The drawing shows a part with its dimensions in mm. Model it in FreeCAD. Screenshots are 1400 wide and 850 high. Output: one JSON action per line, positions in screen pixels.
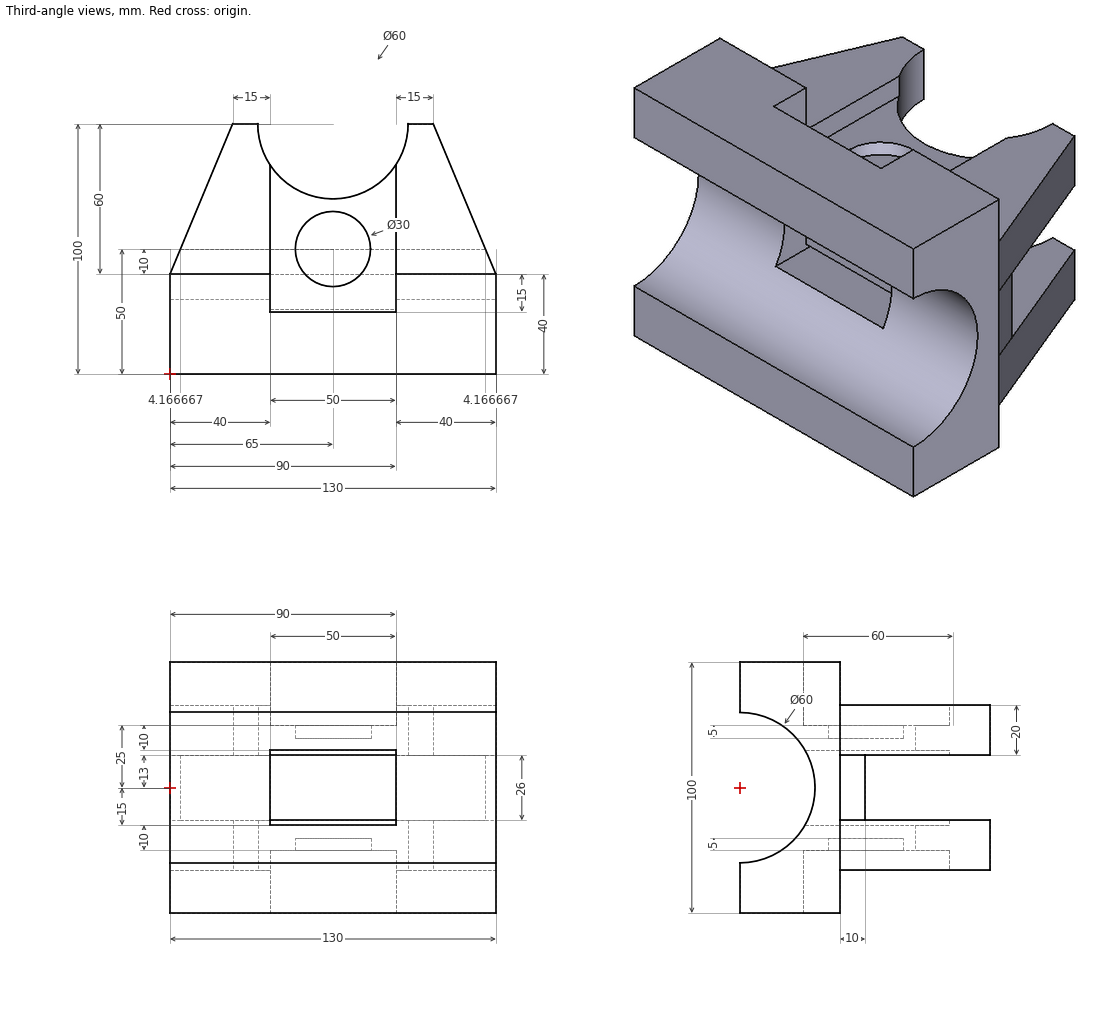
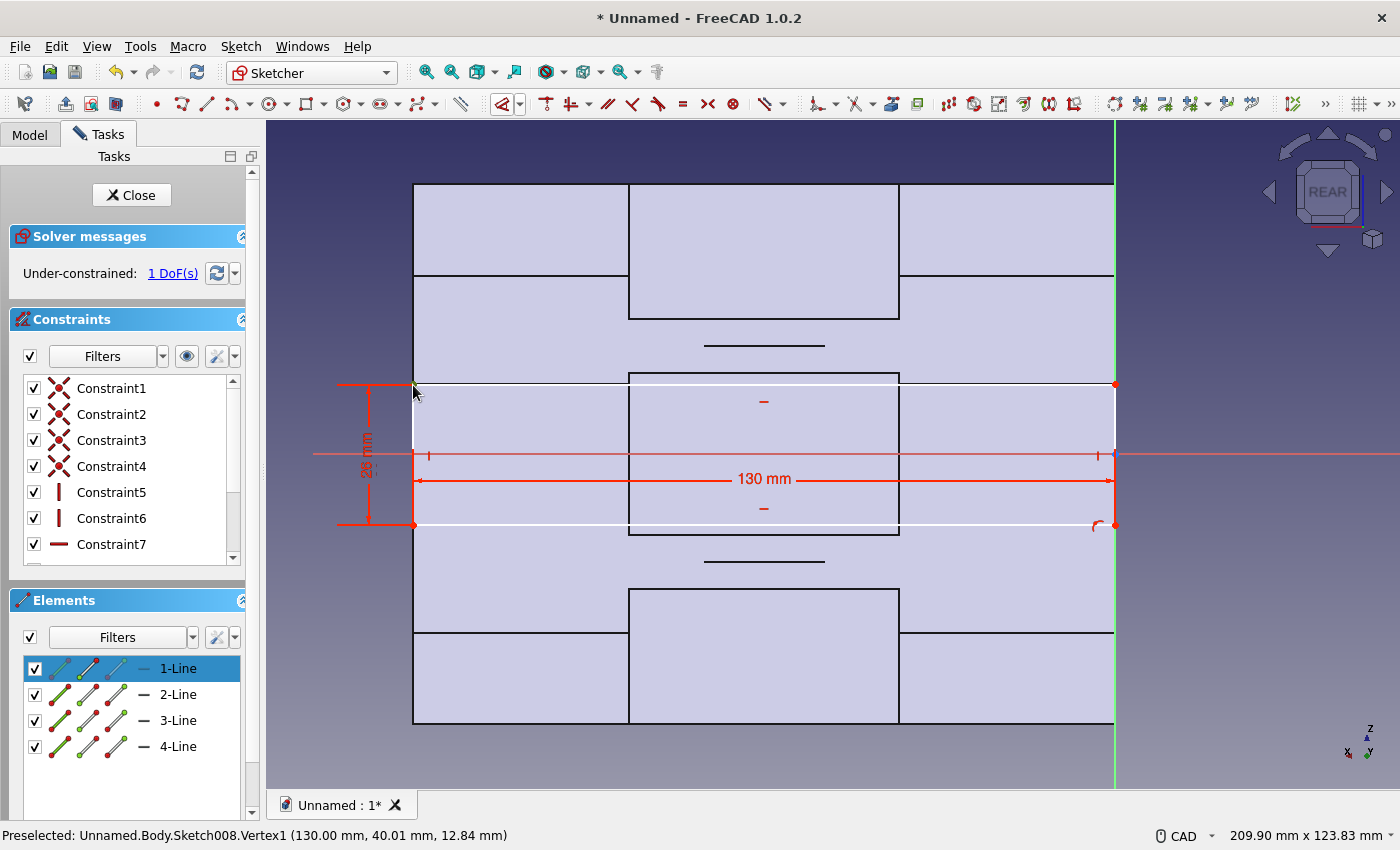
{"action": "left_click", "coordinate": [520, 104]}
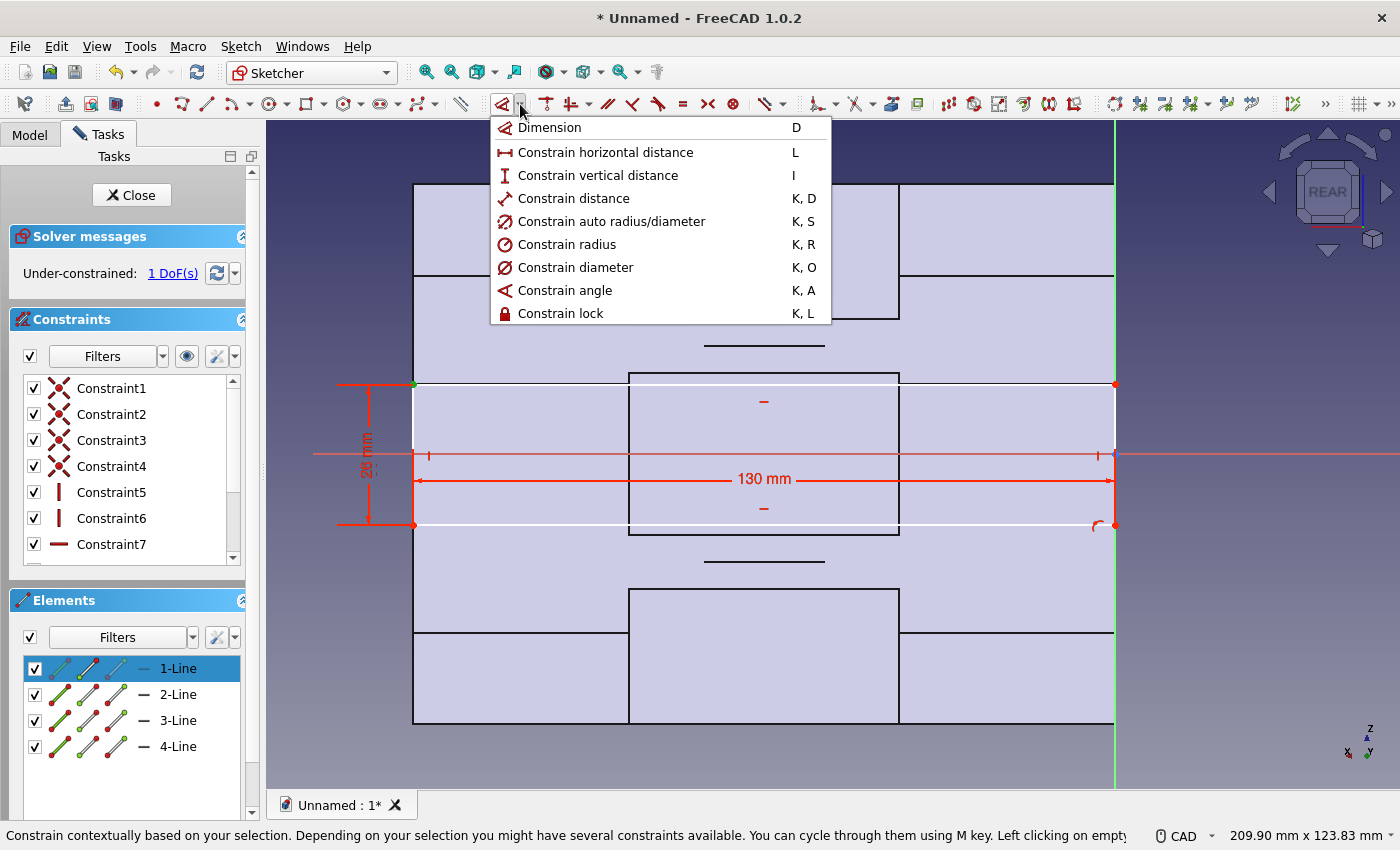
{"action": "left_click", "coordinate": [661, 176]}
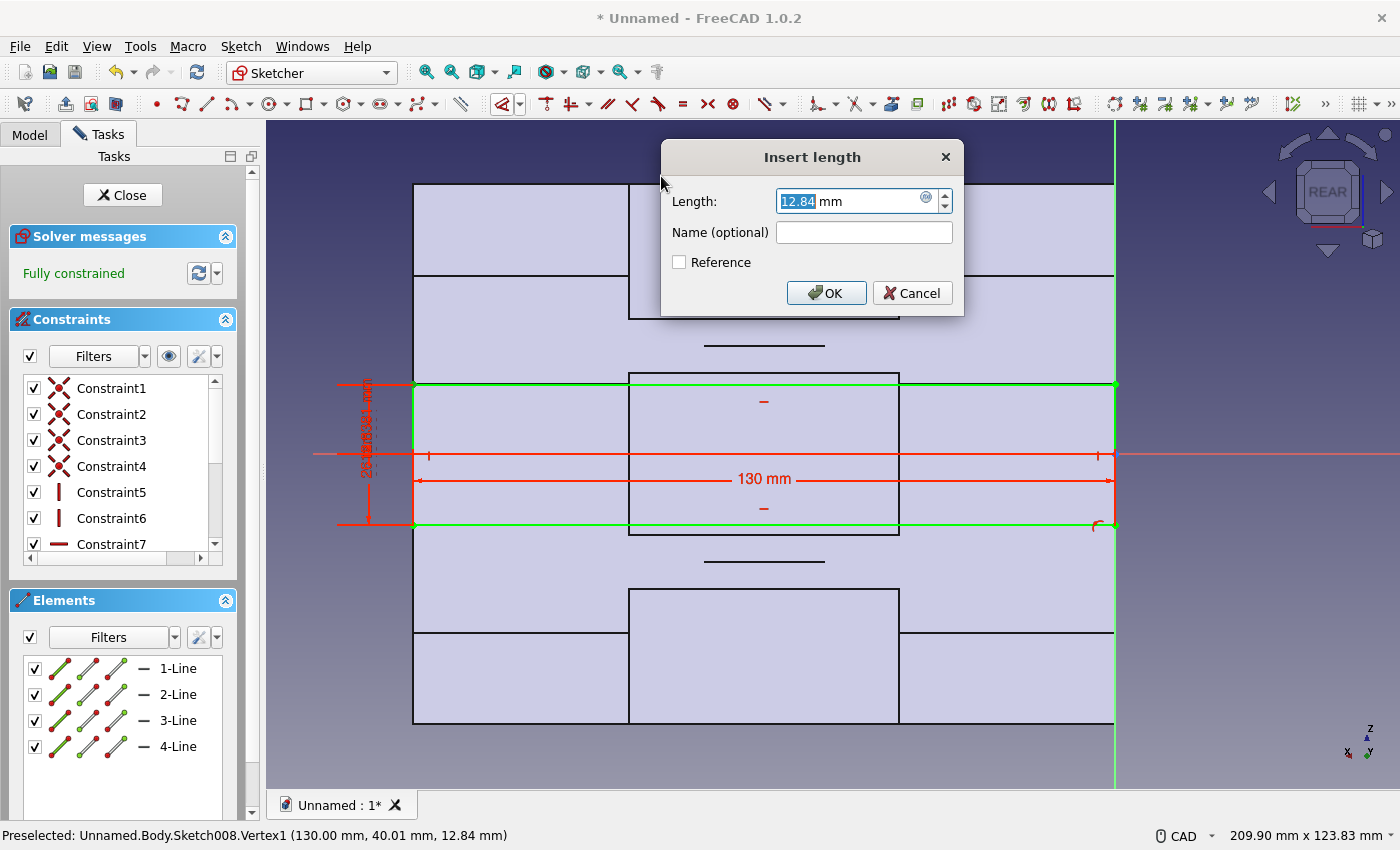
{"action": "type", "text": "13"}
{"action": "key", "text": "Return"}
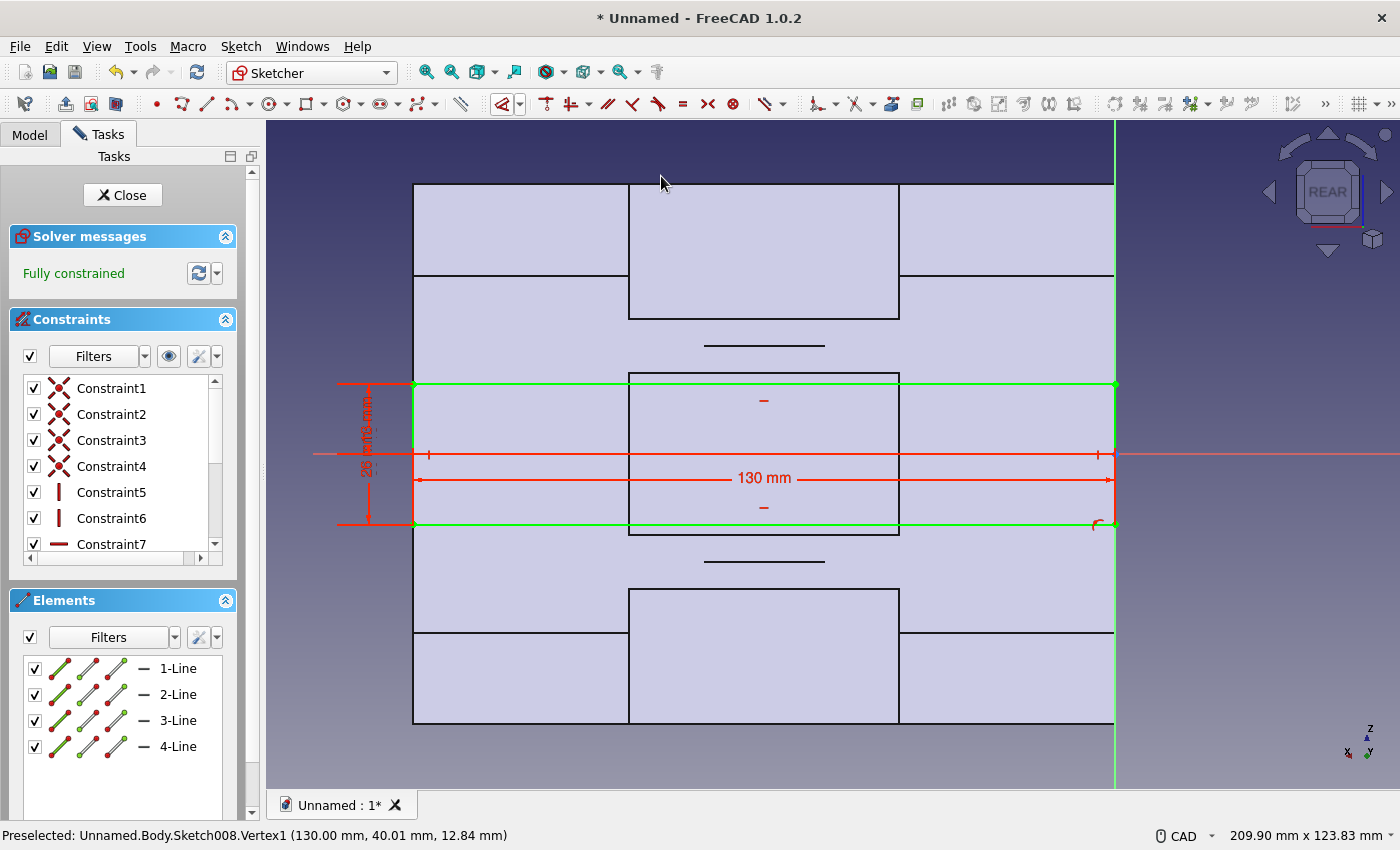
{"action": "left_click", "coordinate": [123, 195]}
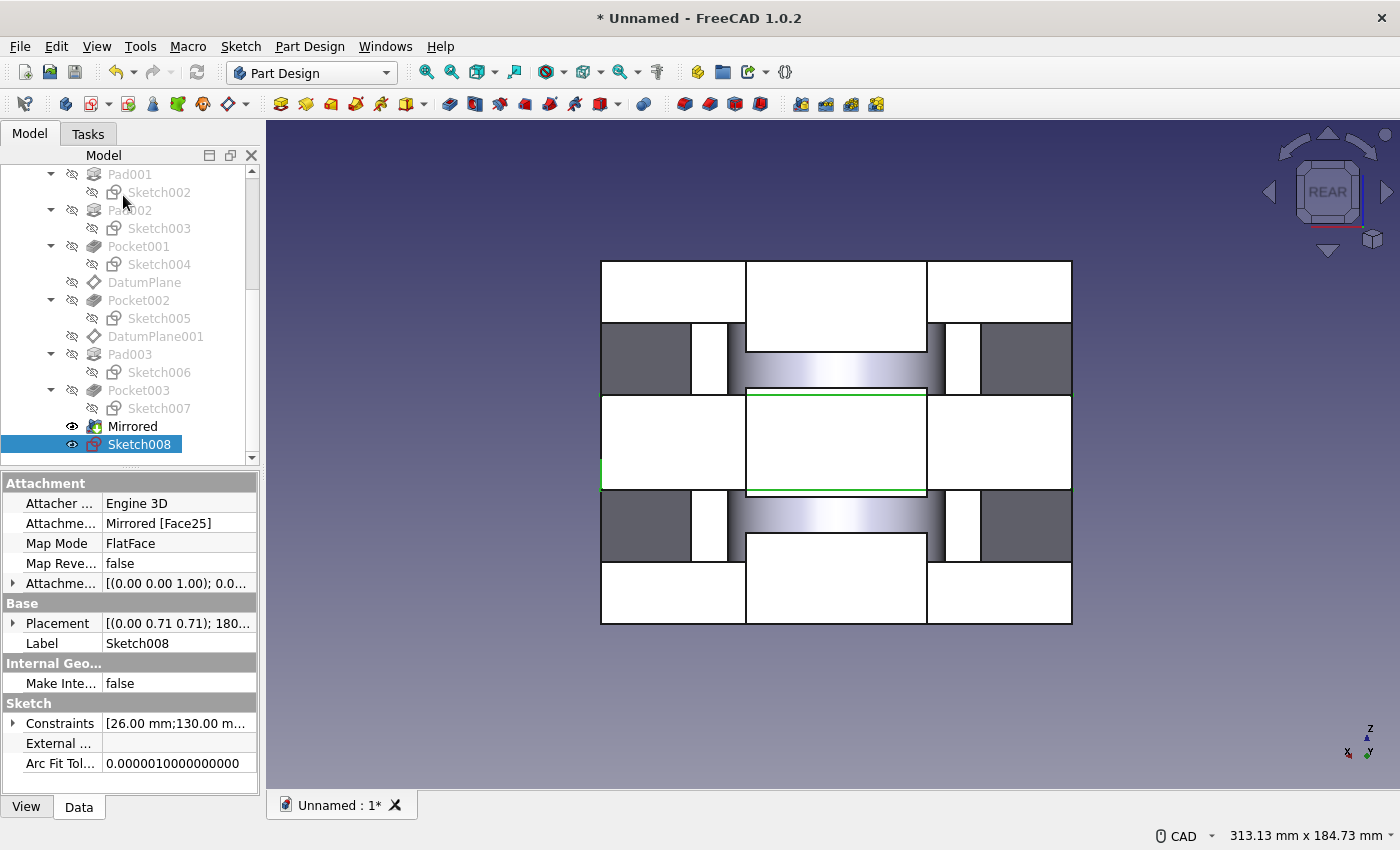
{"action": "left_click", "coordinate": [281, 104]}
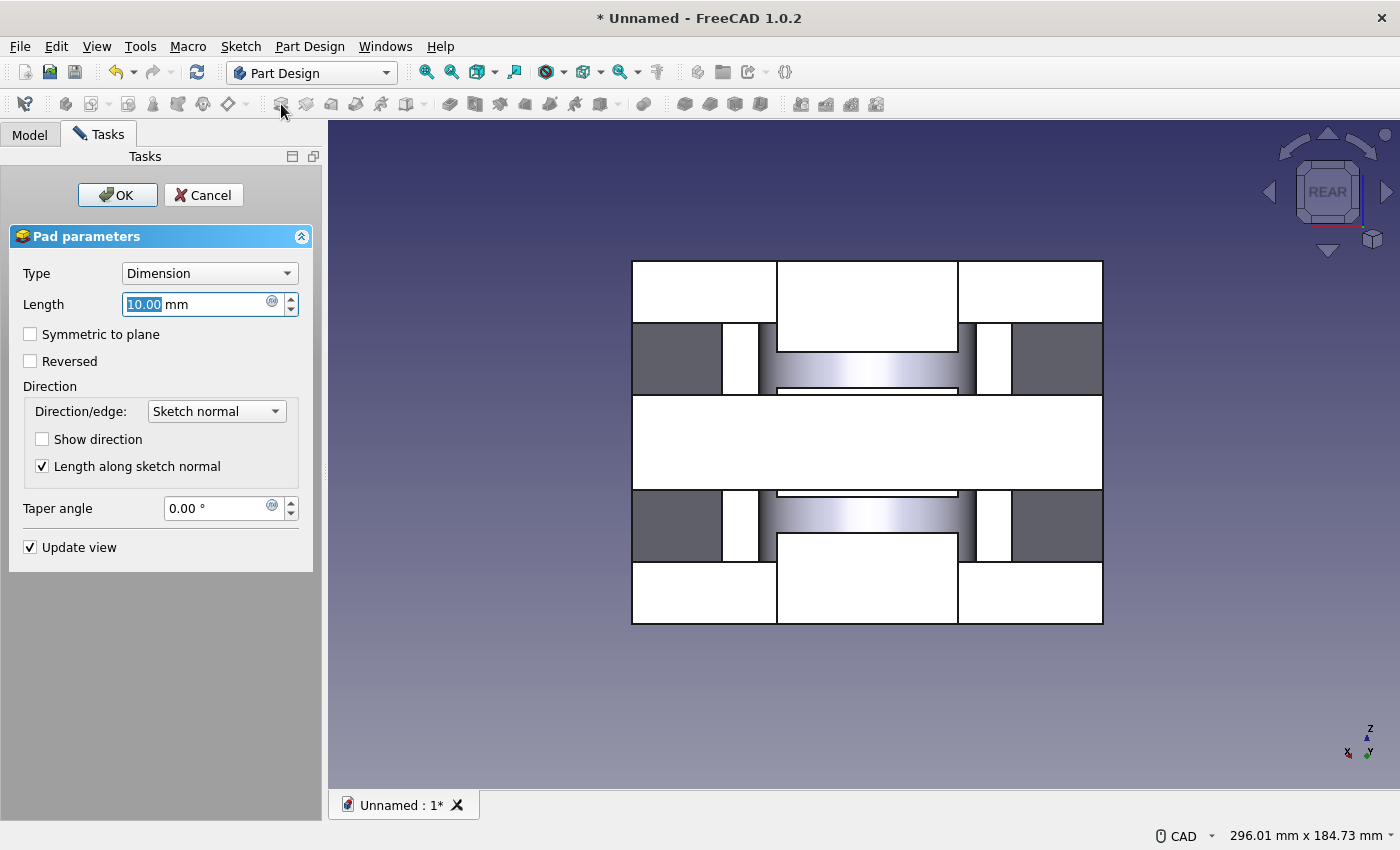
{"action": "type", "text": "10"}
{"action": "key", "text": "Tab"}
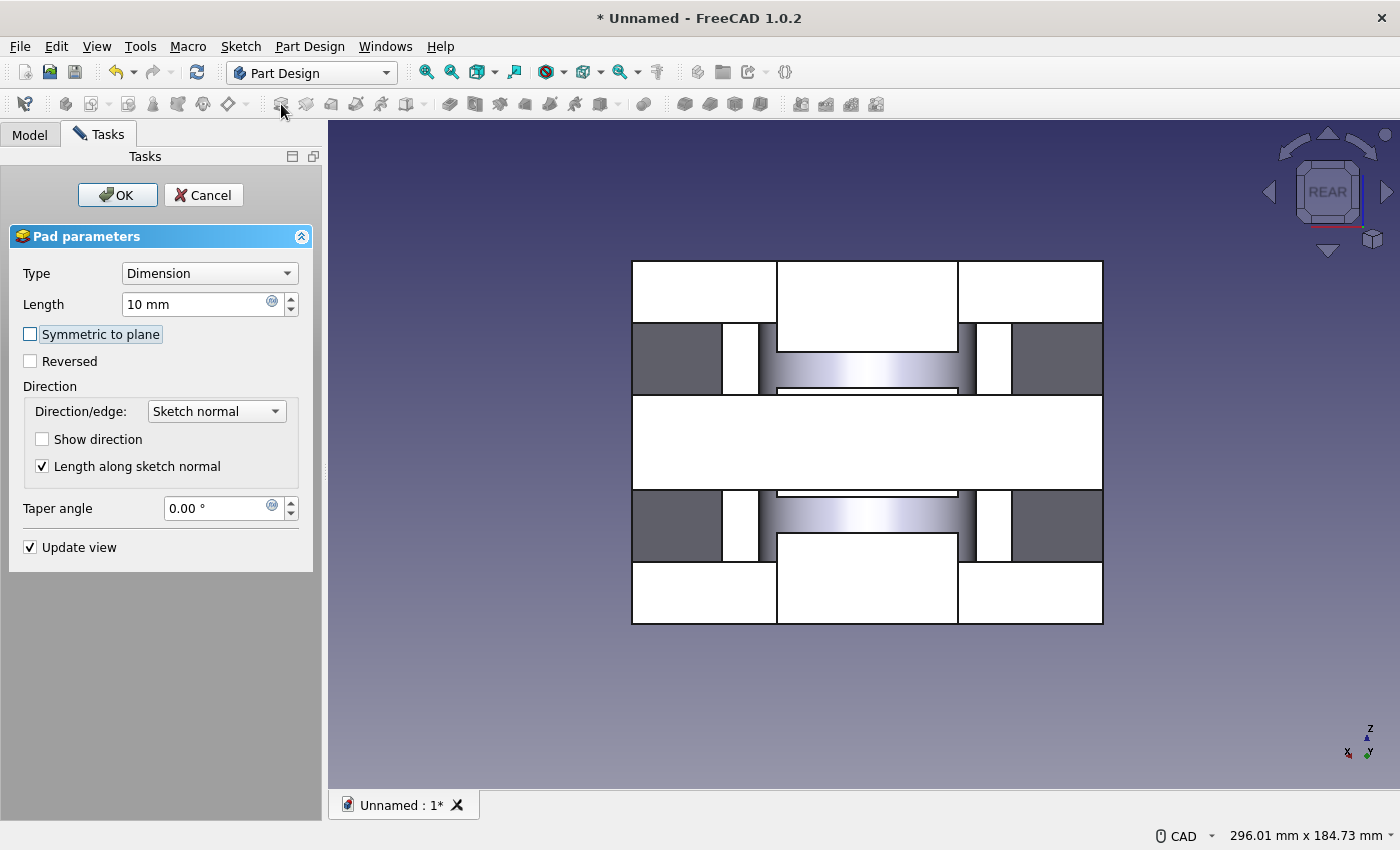
{"action": "left_click", "coordinate": [118, 195]}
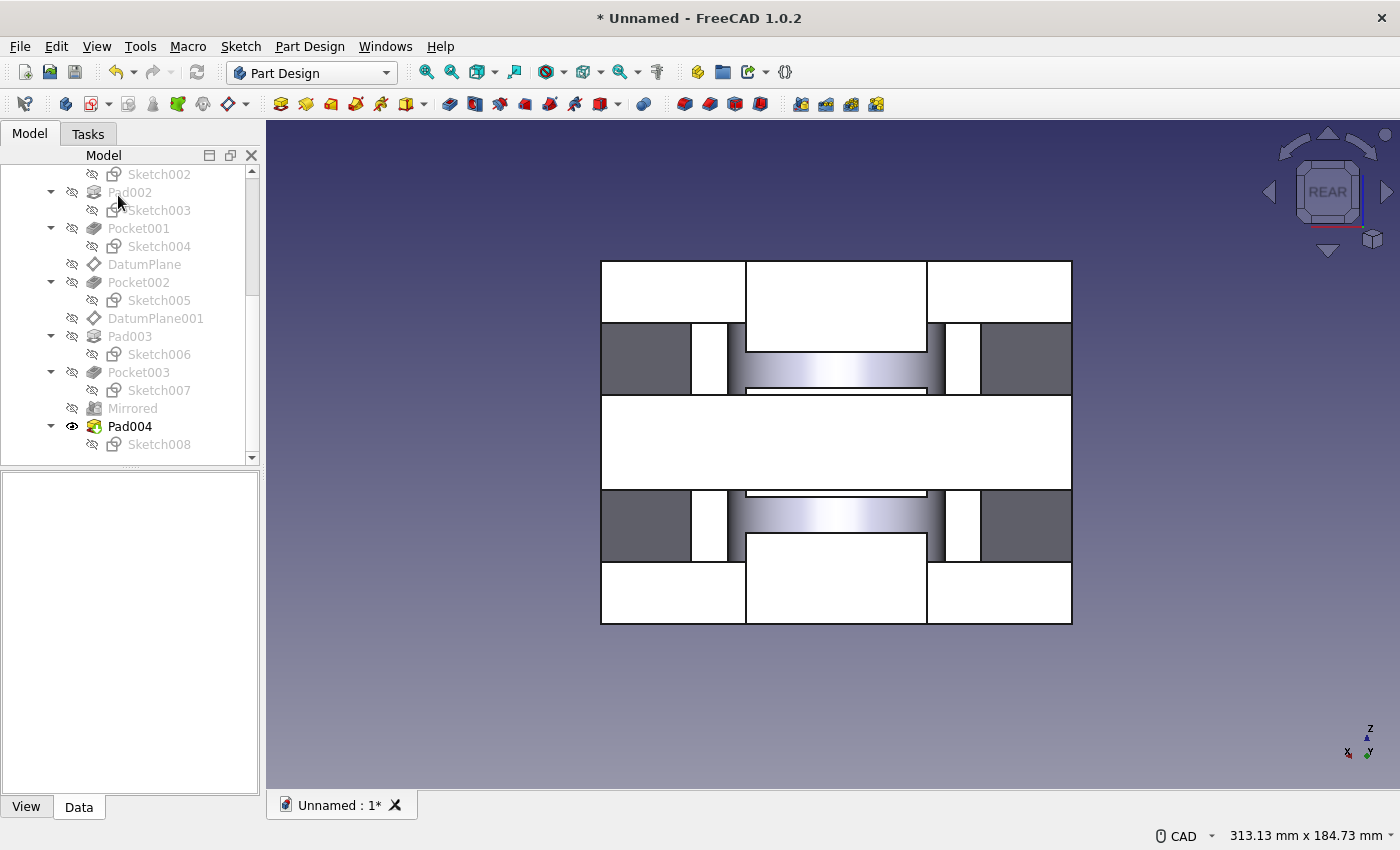
{"action": "key", "text": "0"}